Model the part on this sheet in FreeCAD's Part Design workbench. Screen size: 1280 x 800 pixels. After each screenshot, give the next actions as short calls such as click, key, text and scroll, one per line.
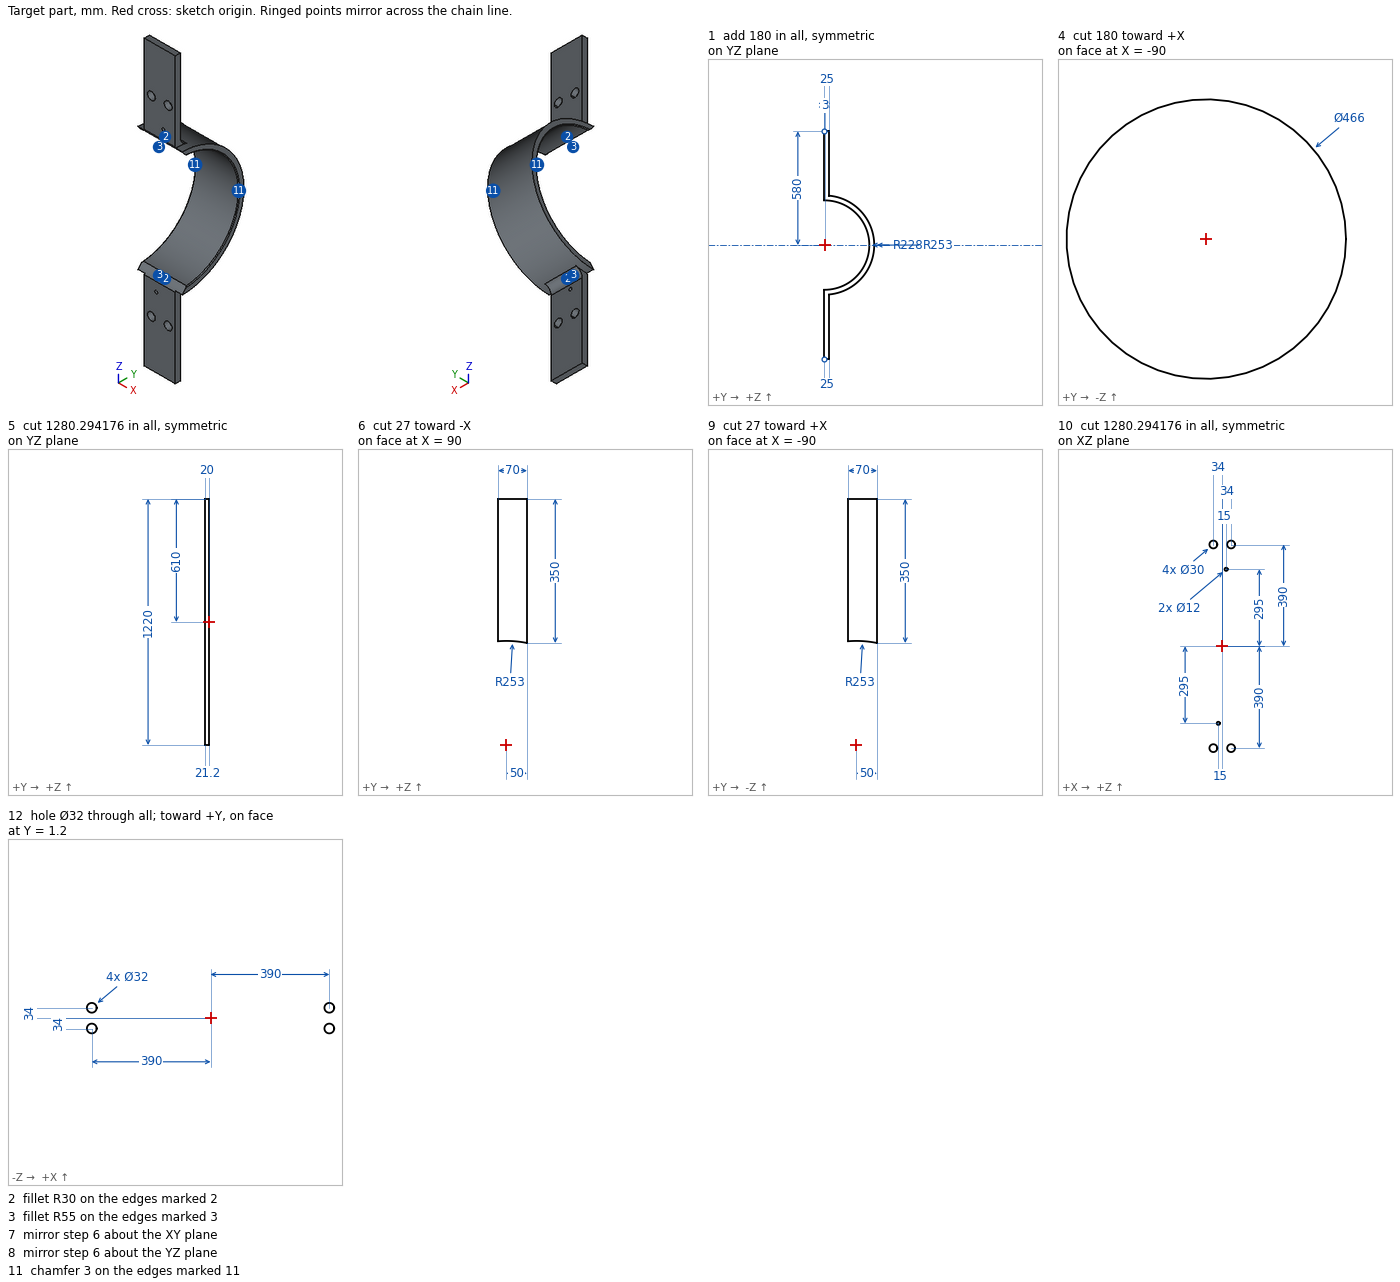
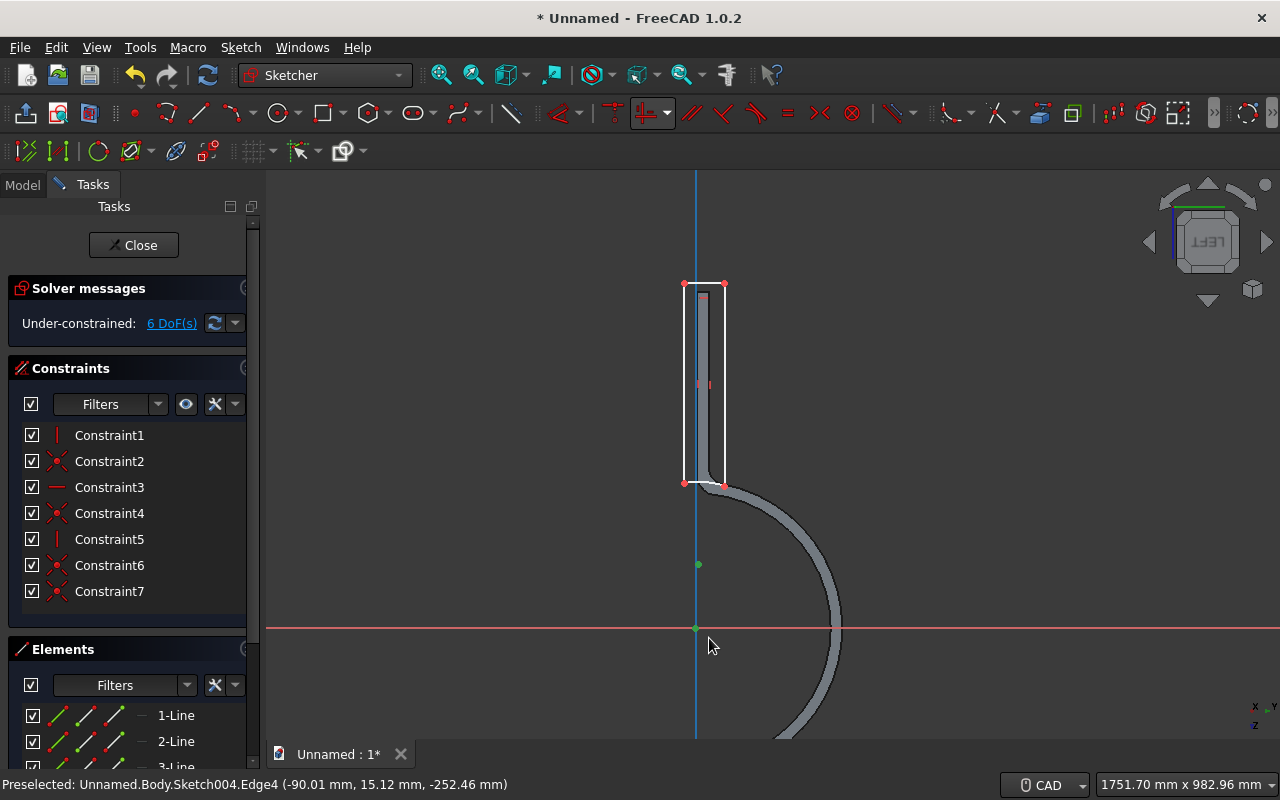
click(614, 114)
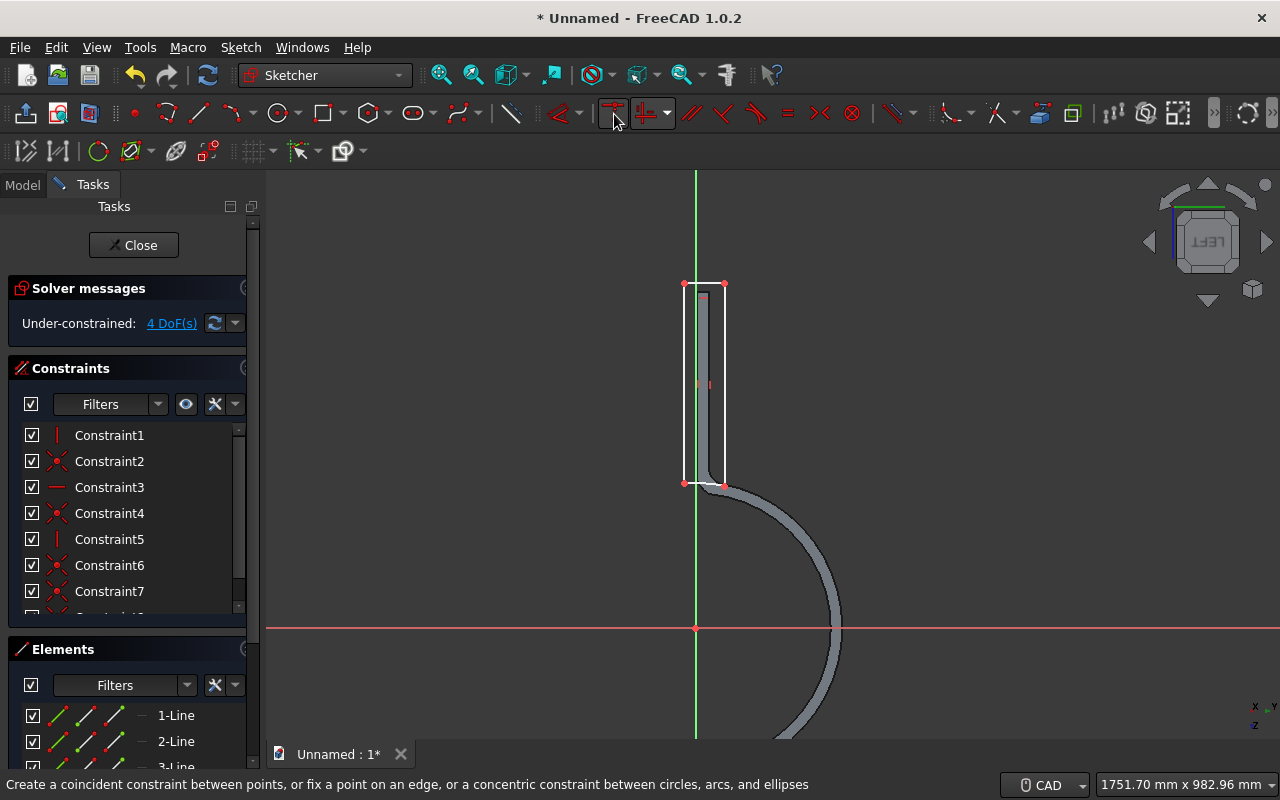
click(558, 114)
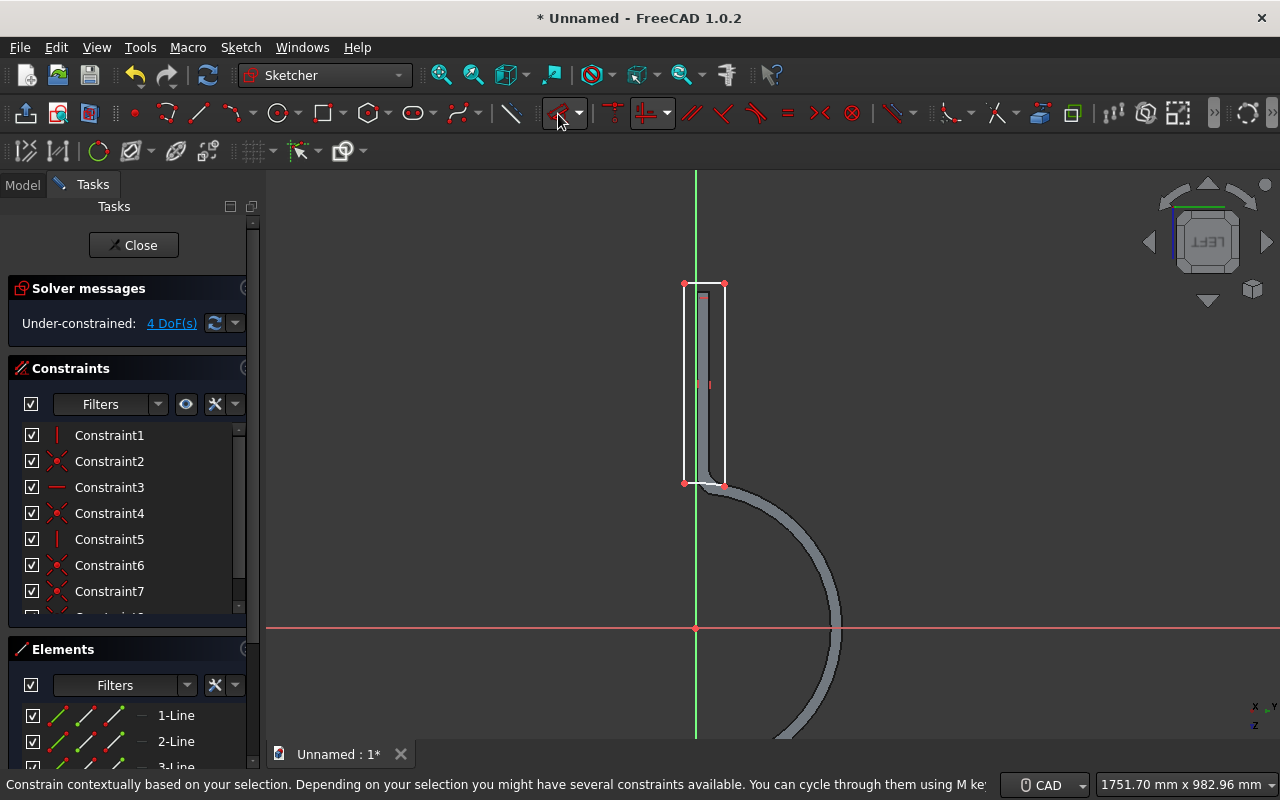
click(713, 484)
click(799, 484)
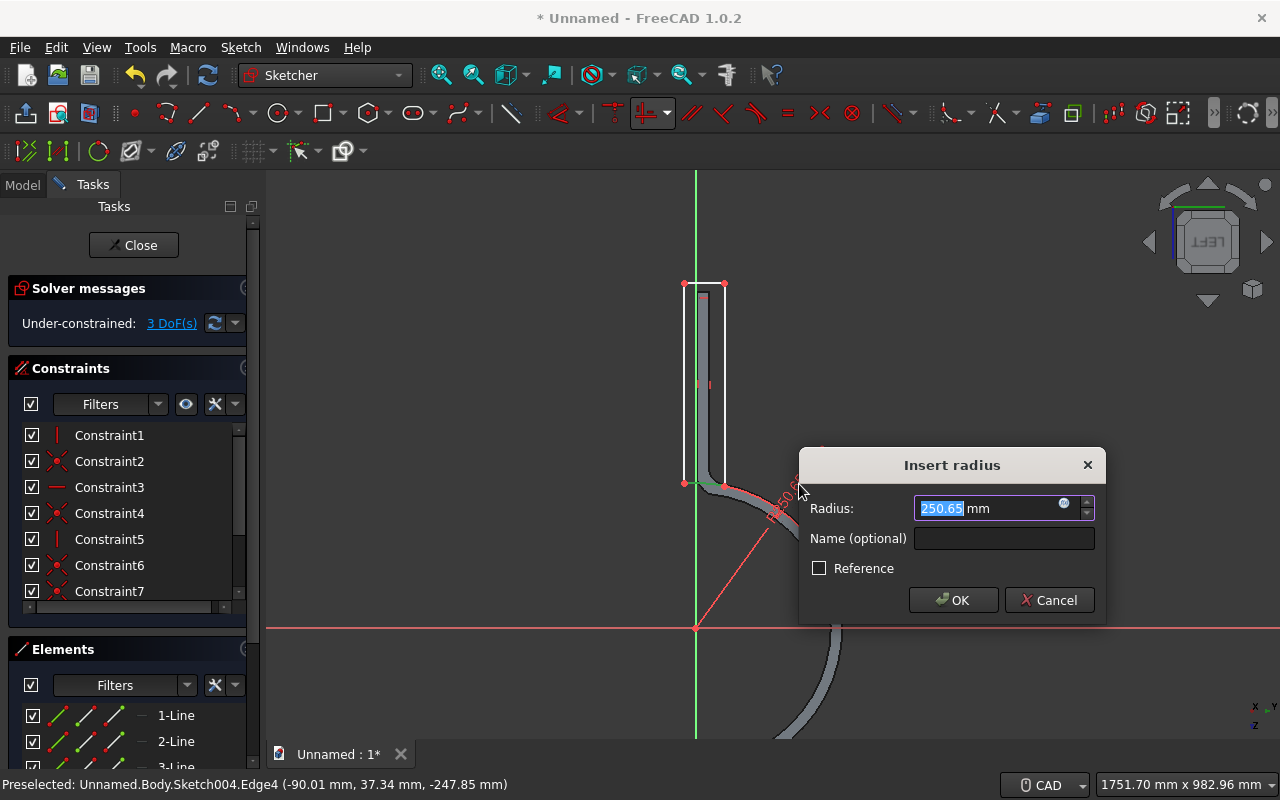
text(253)
key(Return)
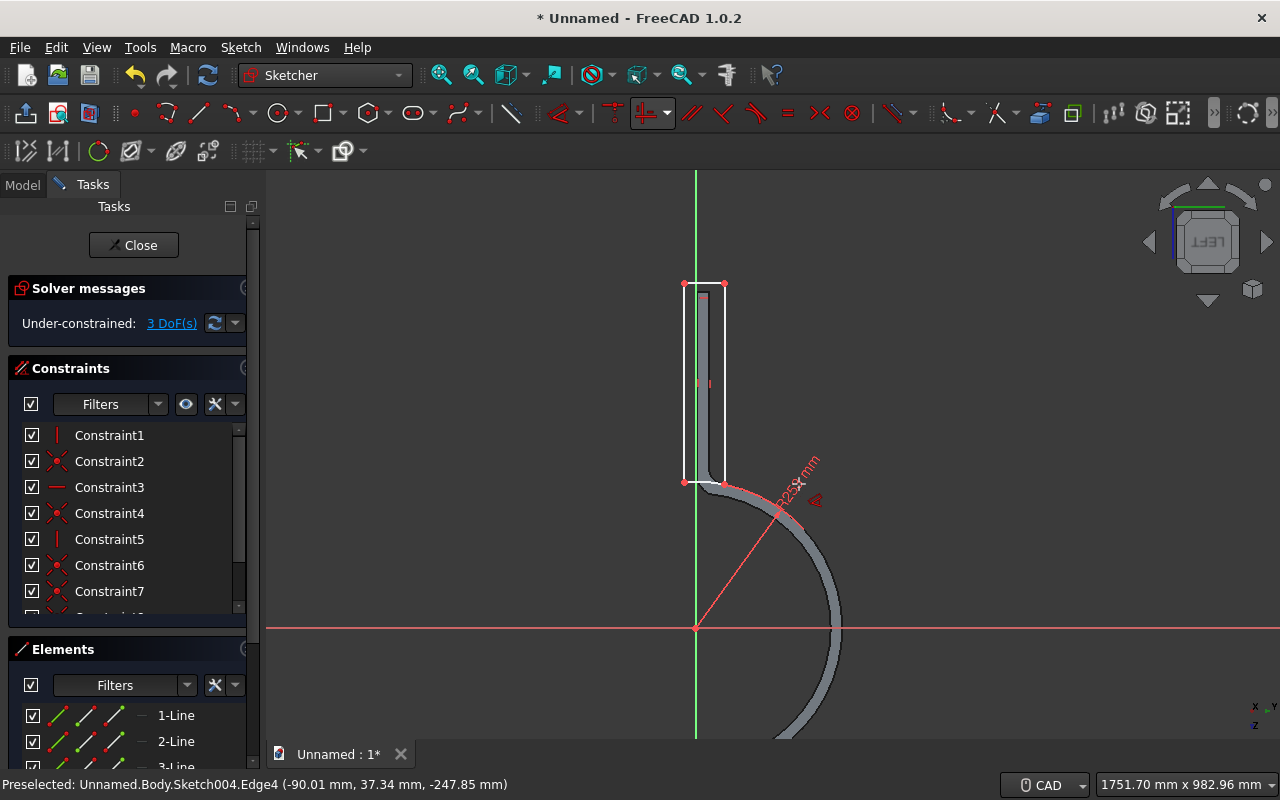
click(713, 283)
click(714, 249)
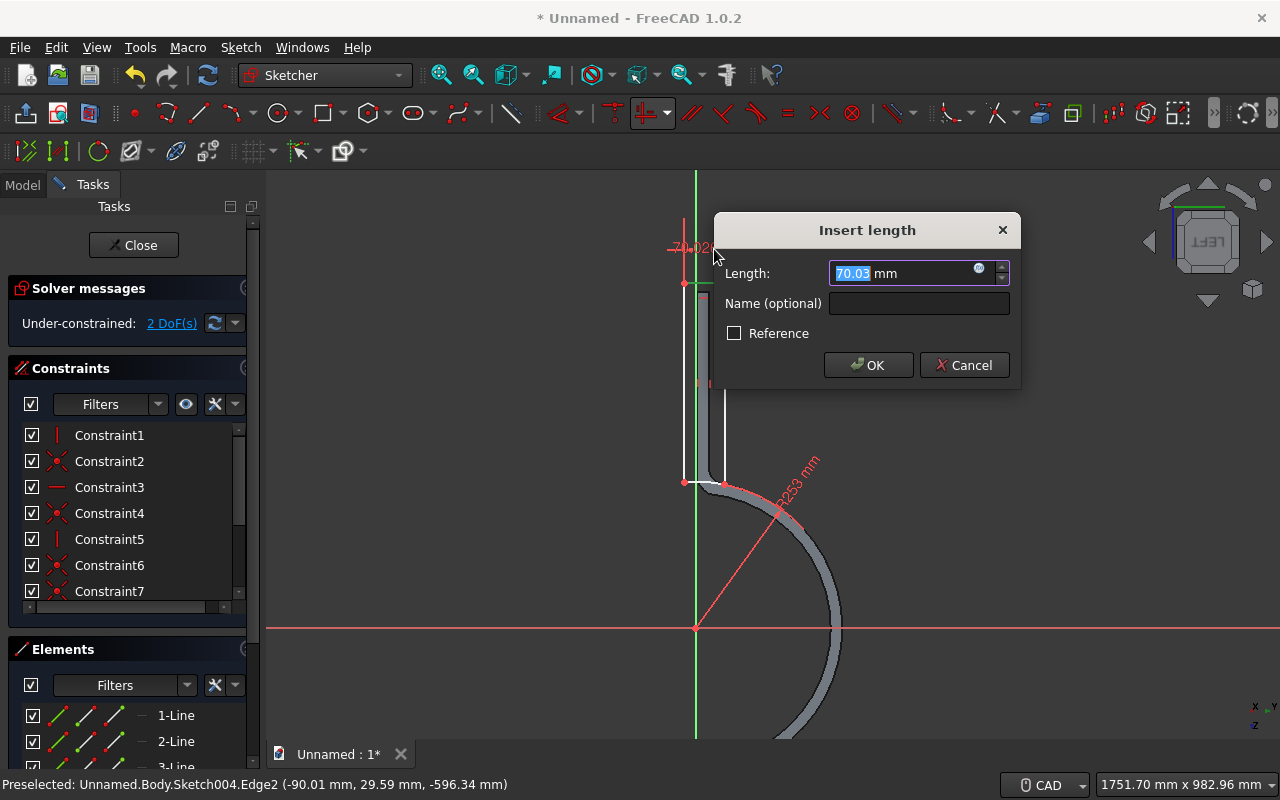
text(70)
key(Return)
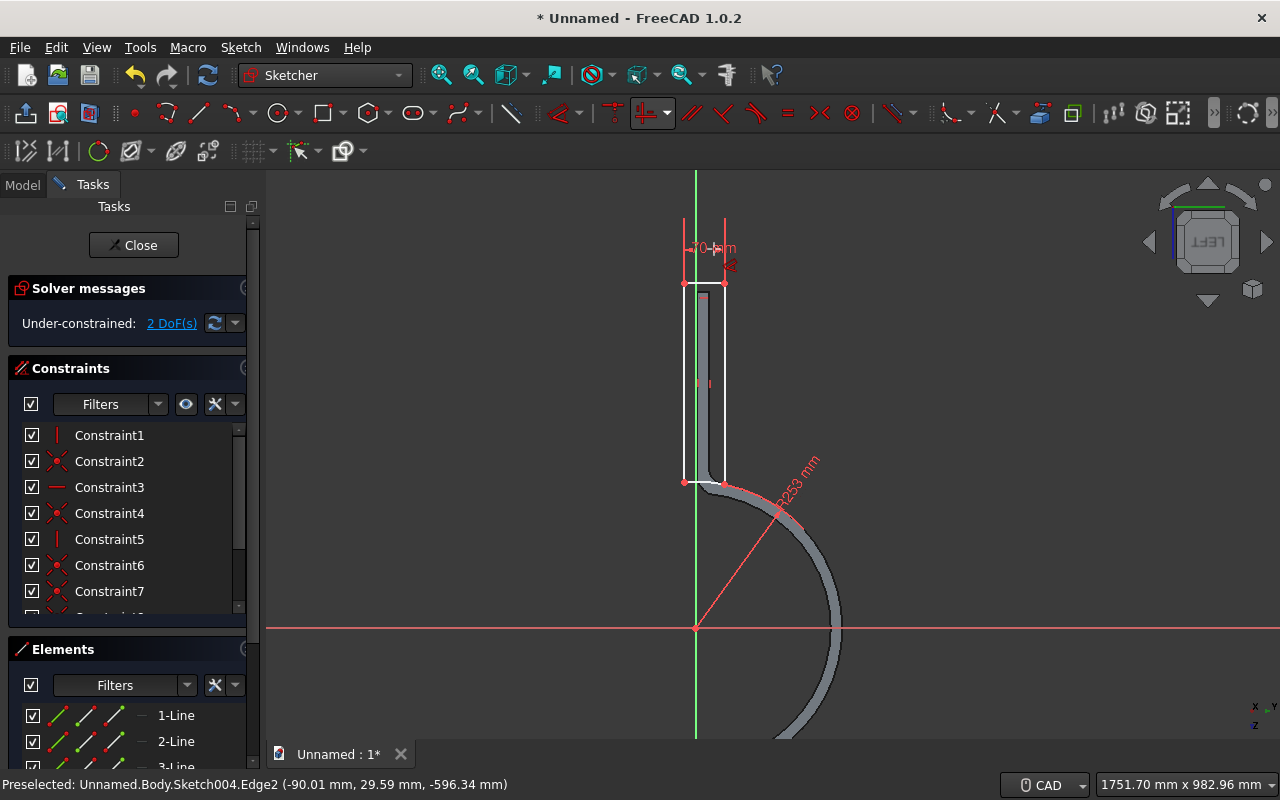
click(725, 424)
click(759, 384)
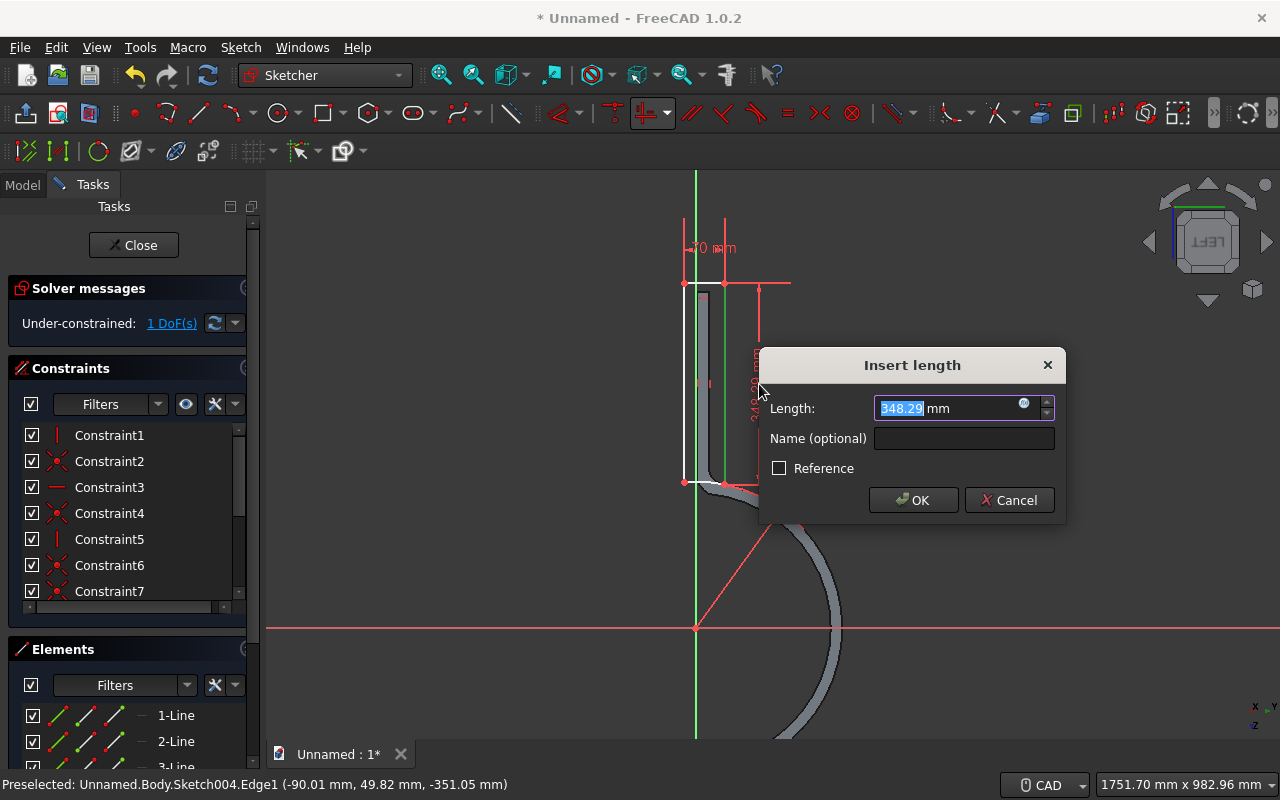
text(350)
key(Return)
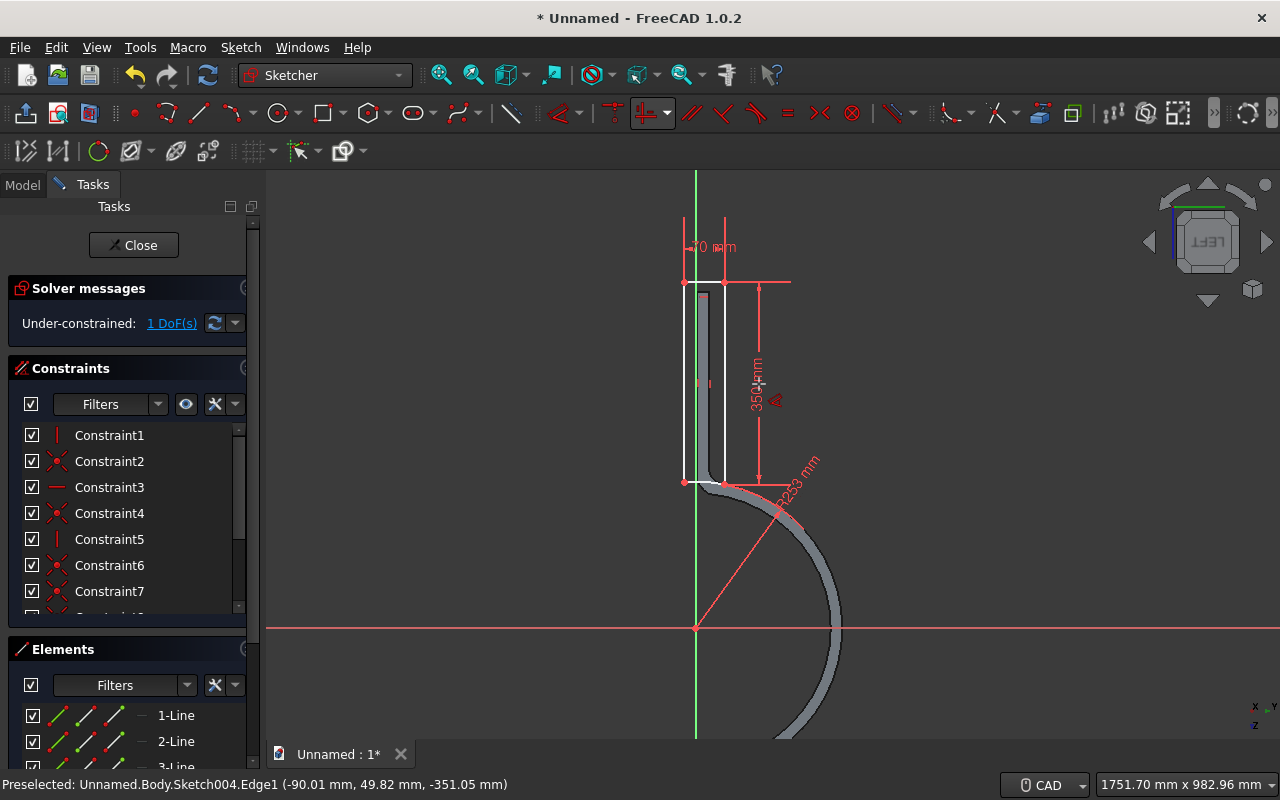
scroll(725, 485, up, 2)